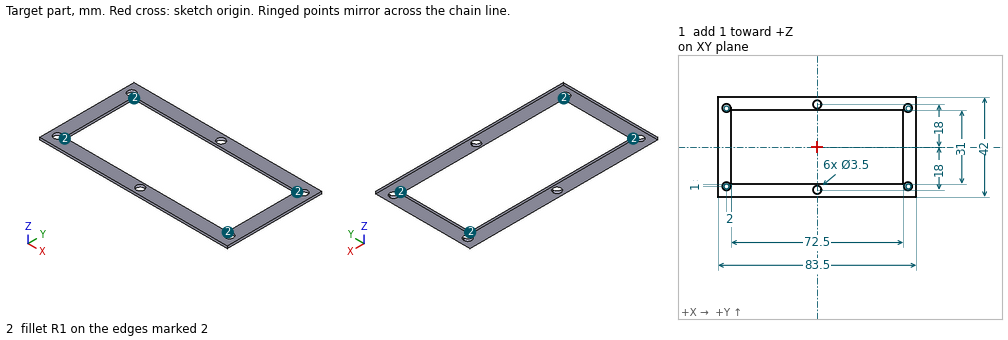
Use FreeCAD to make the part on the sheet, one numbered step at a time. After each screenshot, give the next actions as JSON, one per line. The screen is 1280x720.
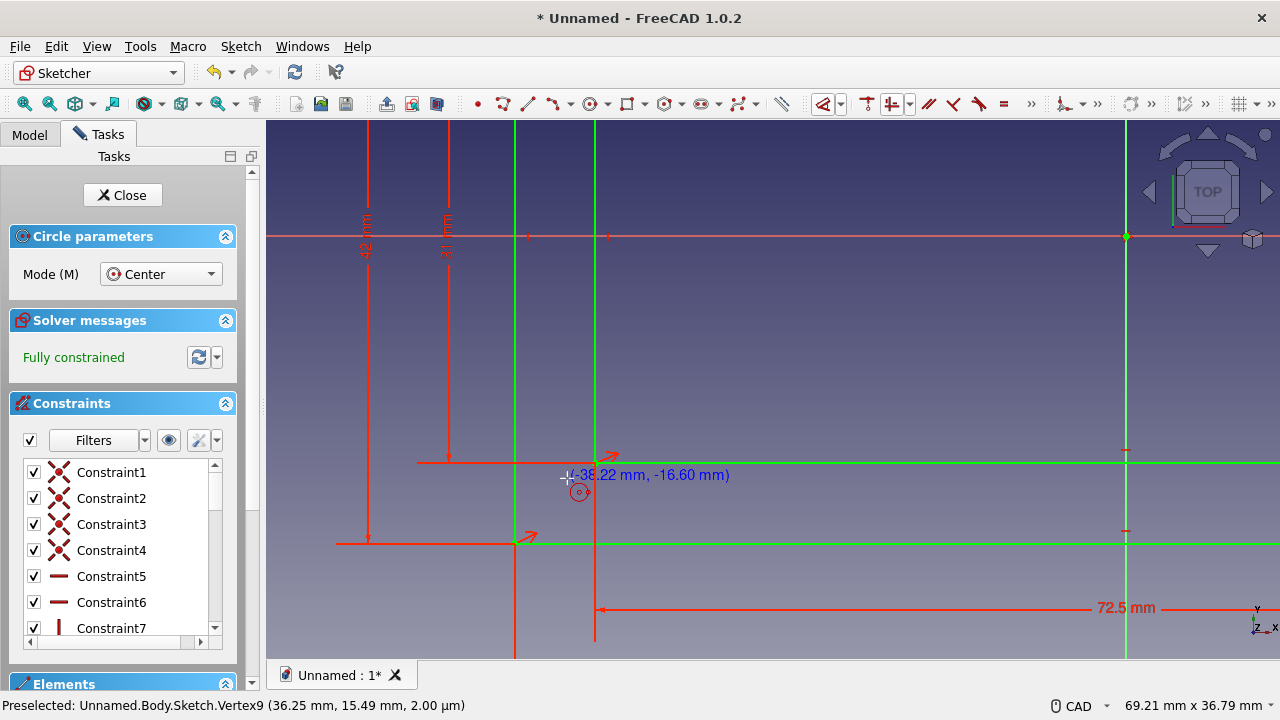
{"action": "left_click", "coordinate": [566, 478]}
{"action": "mouse_move", "coordinate": [548, 460]}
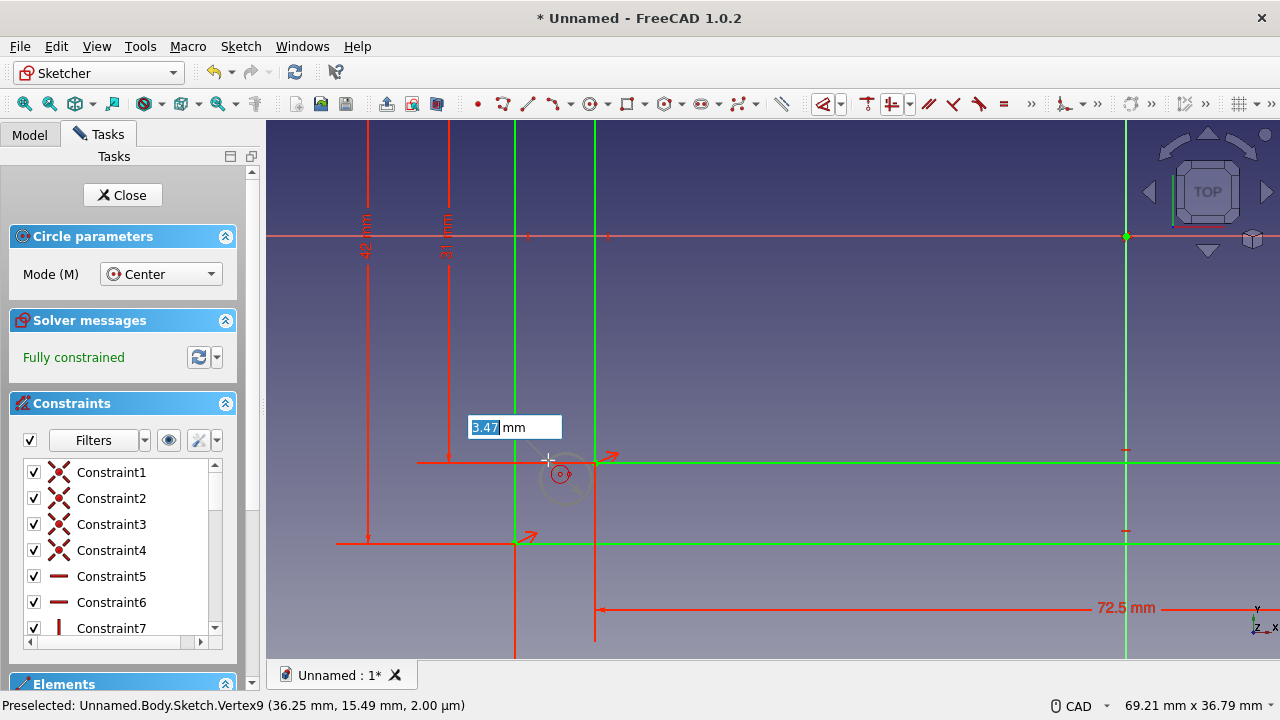
{"action": "type", "text": "3.5"}
{"action": "key", "text": "Return"}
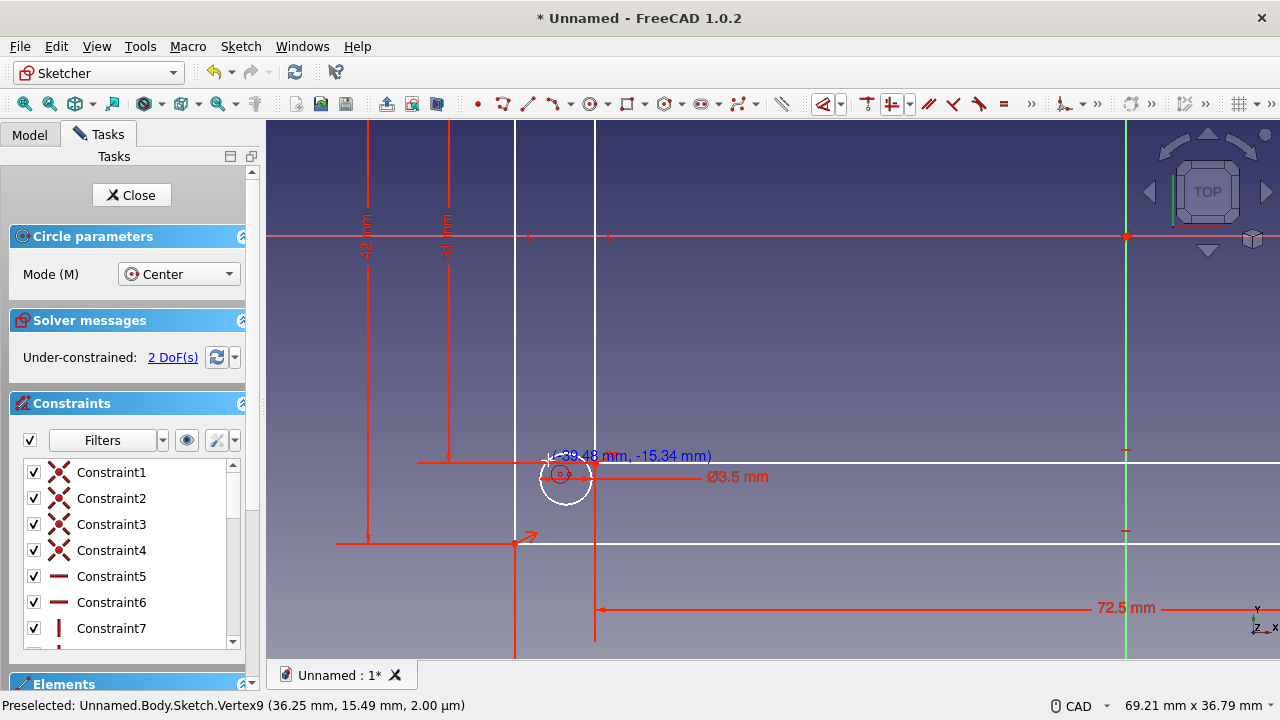
{"action": "scroll", "coordinate": [360, 515], "scroll_direction": "down", "scroll_amount": 4}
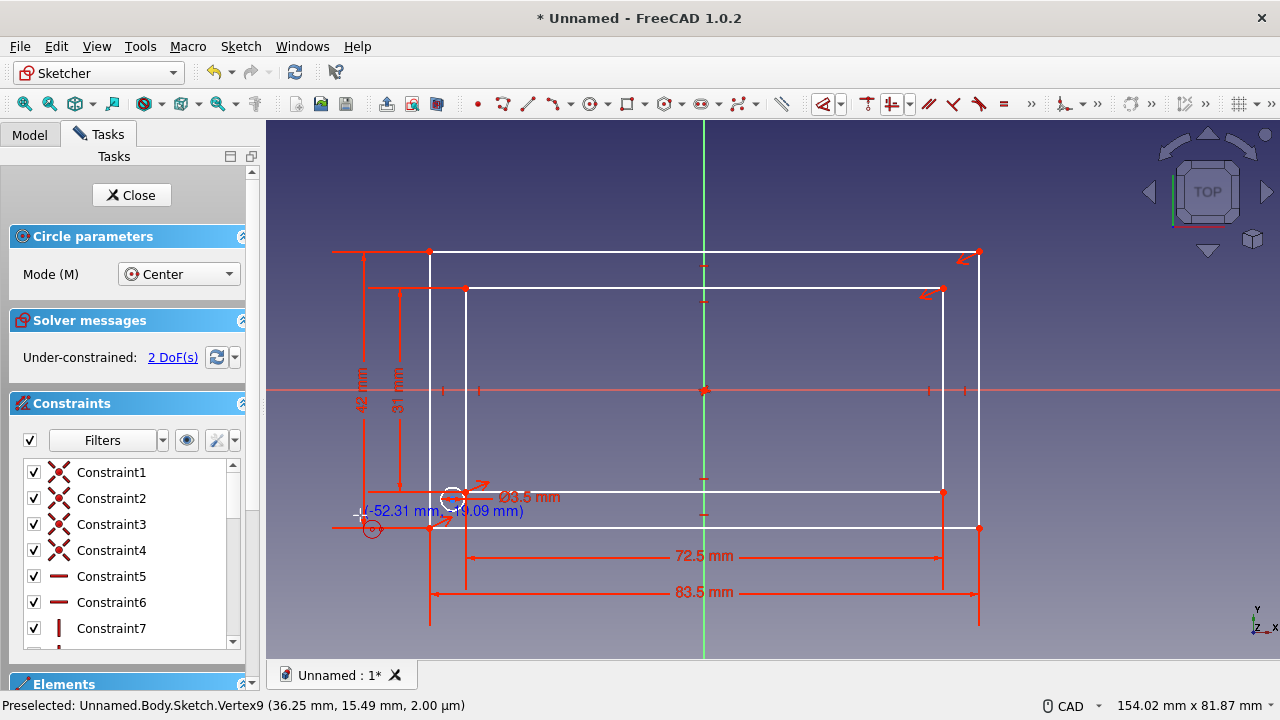
{"action": "scroll", "coordinate": [704, 509], "scroll_direction": "up", "scroll_amount": 4}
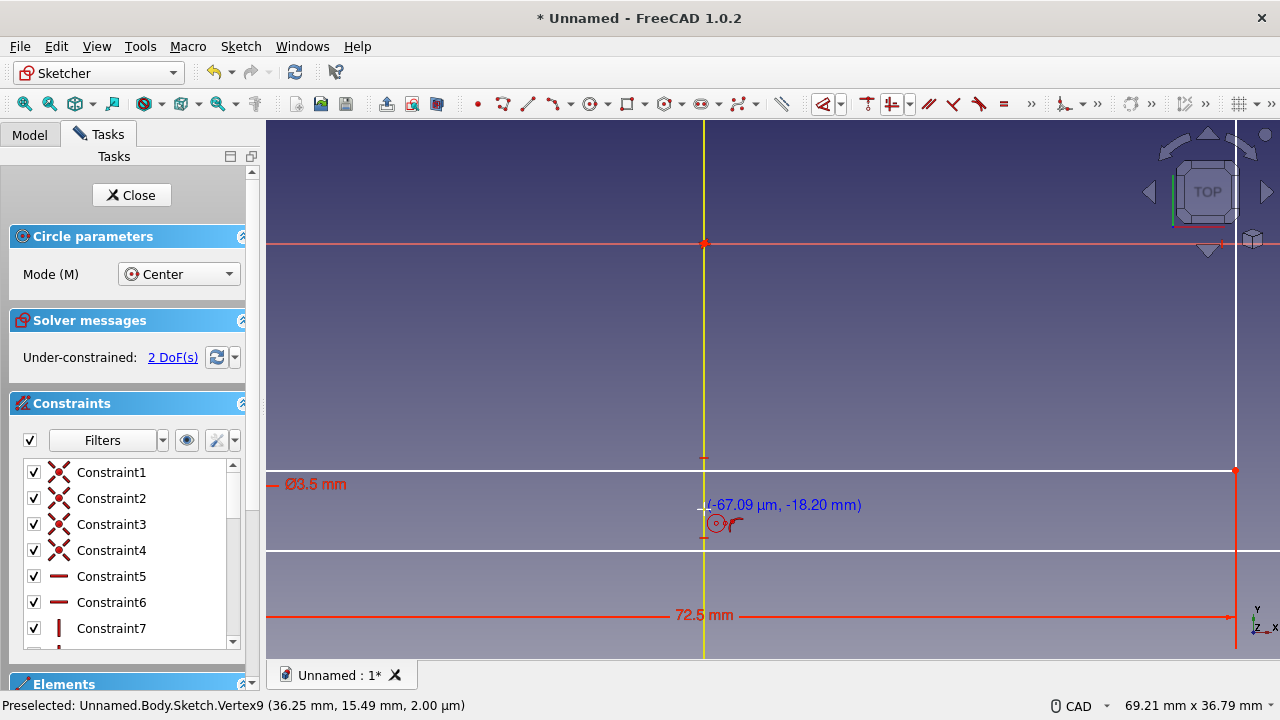
{"action": "left_click", "coordinate": [704, 507]}
{"action": "mouse_move", "coordinate": [723, 489]}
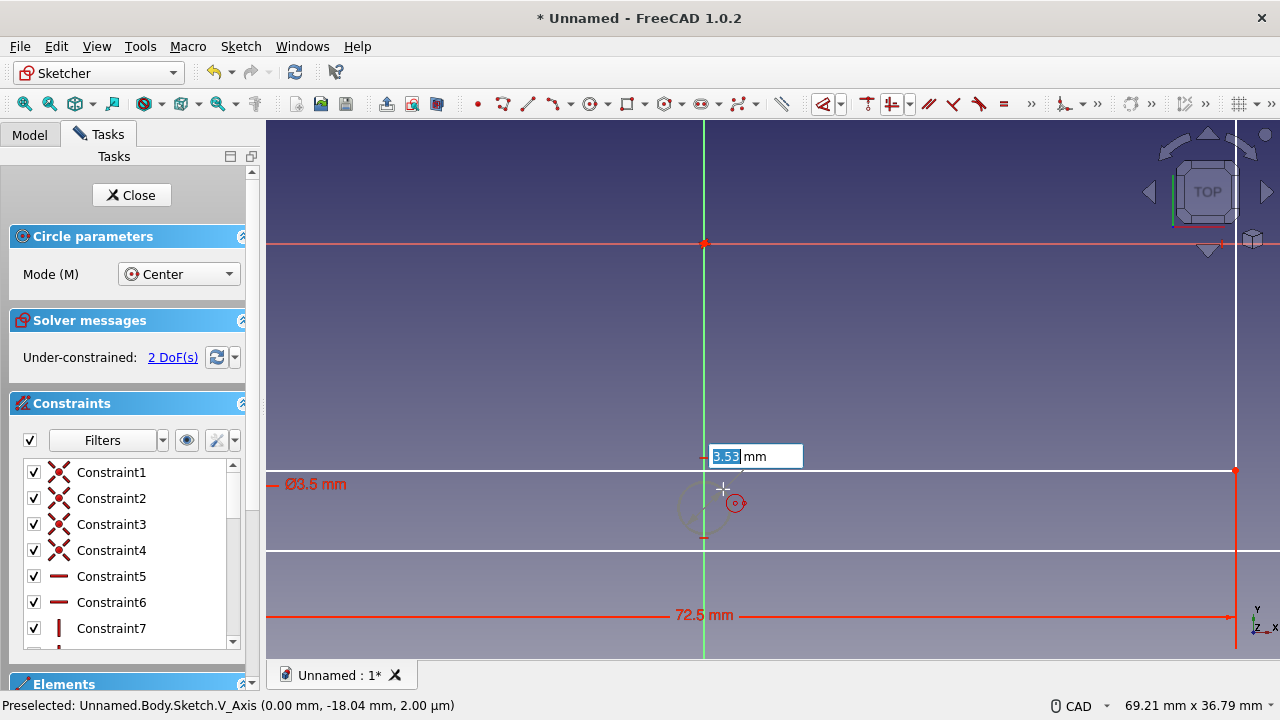
{"action": "type", "text": "3.5"}
{"action": "key", "text": "Return"}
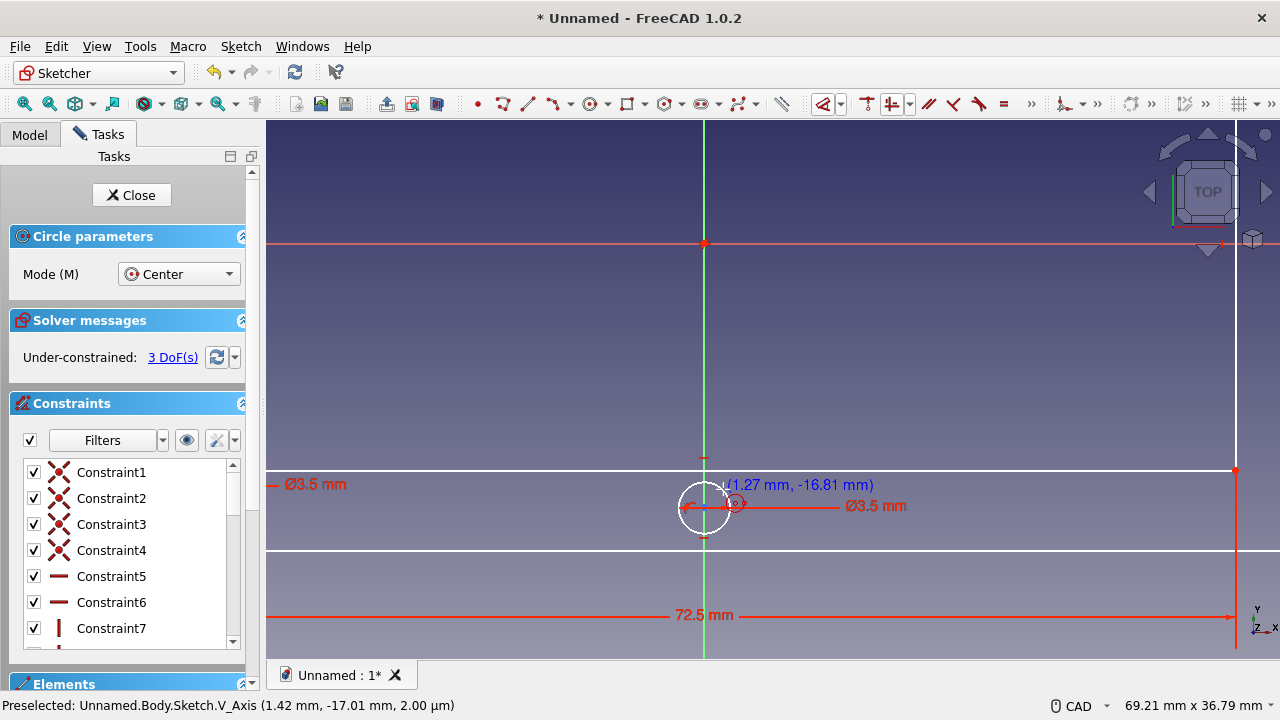
{"action": "scroll", "coordinate": [705, 509], "scroll_direction": "down", "scroll_amount": 4}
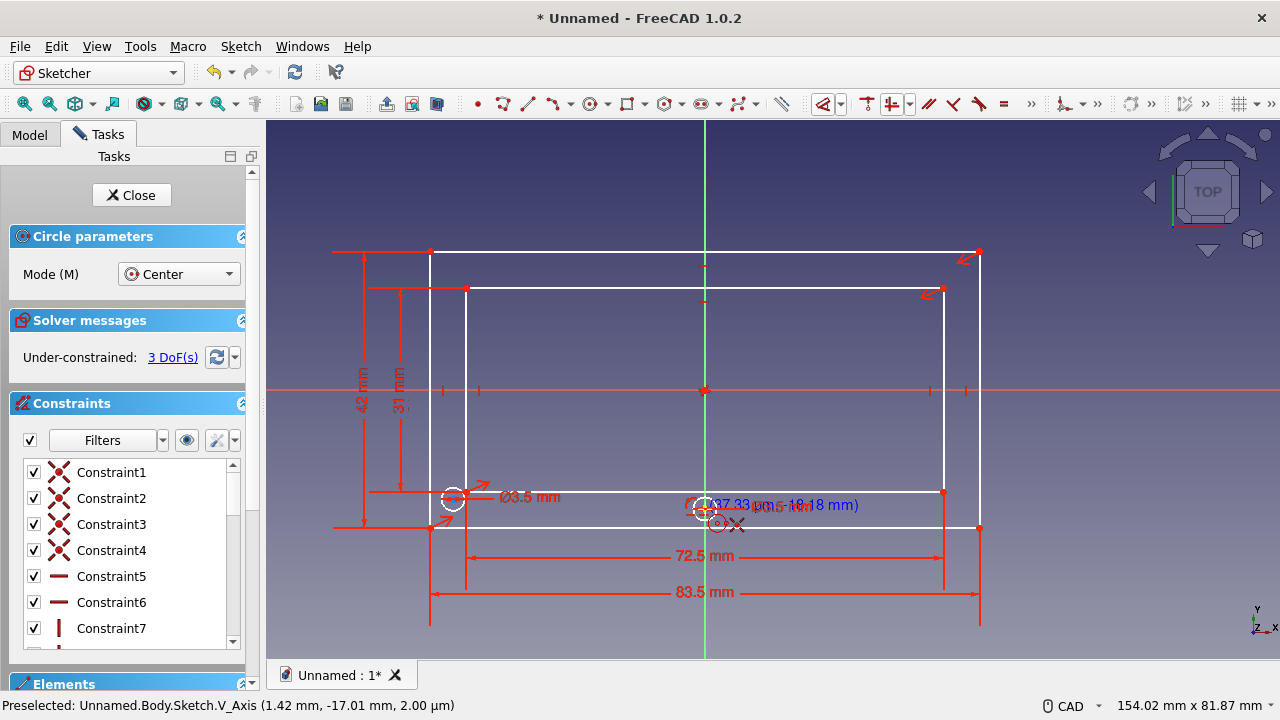
{"action": "scroll", "coordinate": [957, 499], "scroll_direction": "up", "scroll_amount": 4}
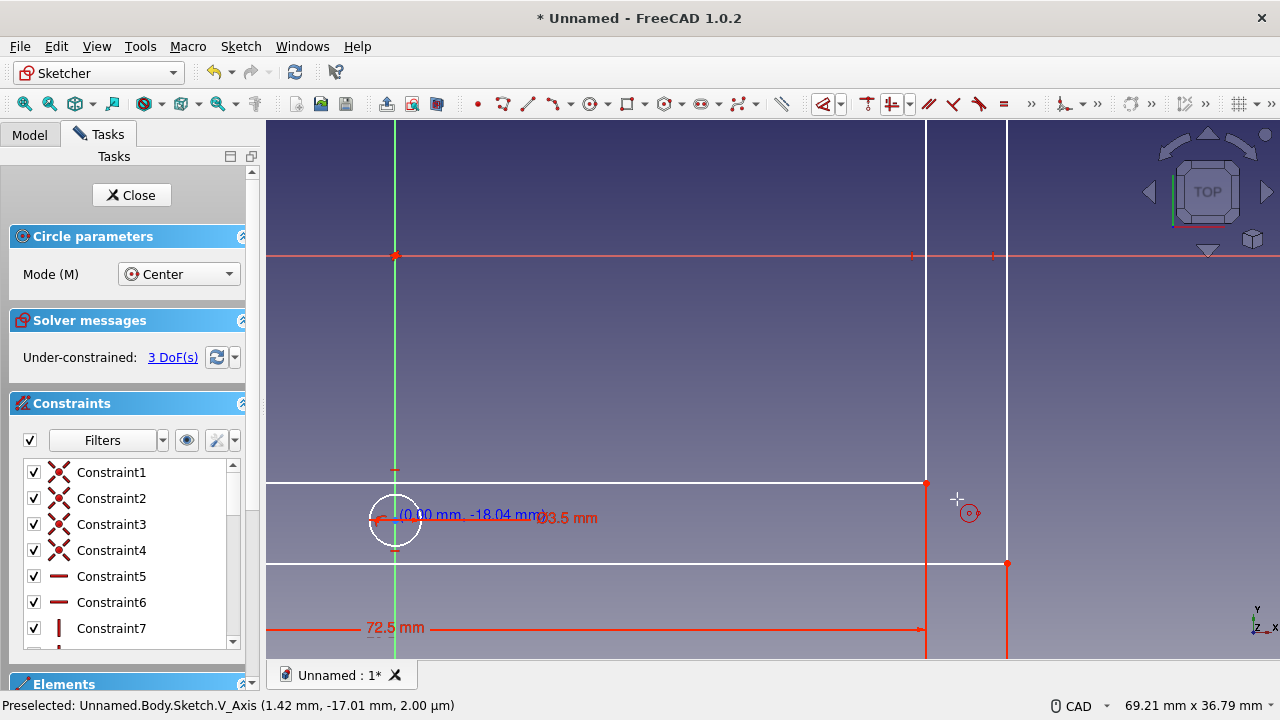
{"action": "left_click", "coordinate": [956, 498]}
{"action": "mouse_move", "coordinate": [974, 480]}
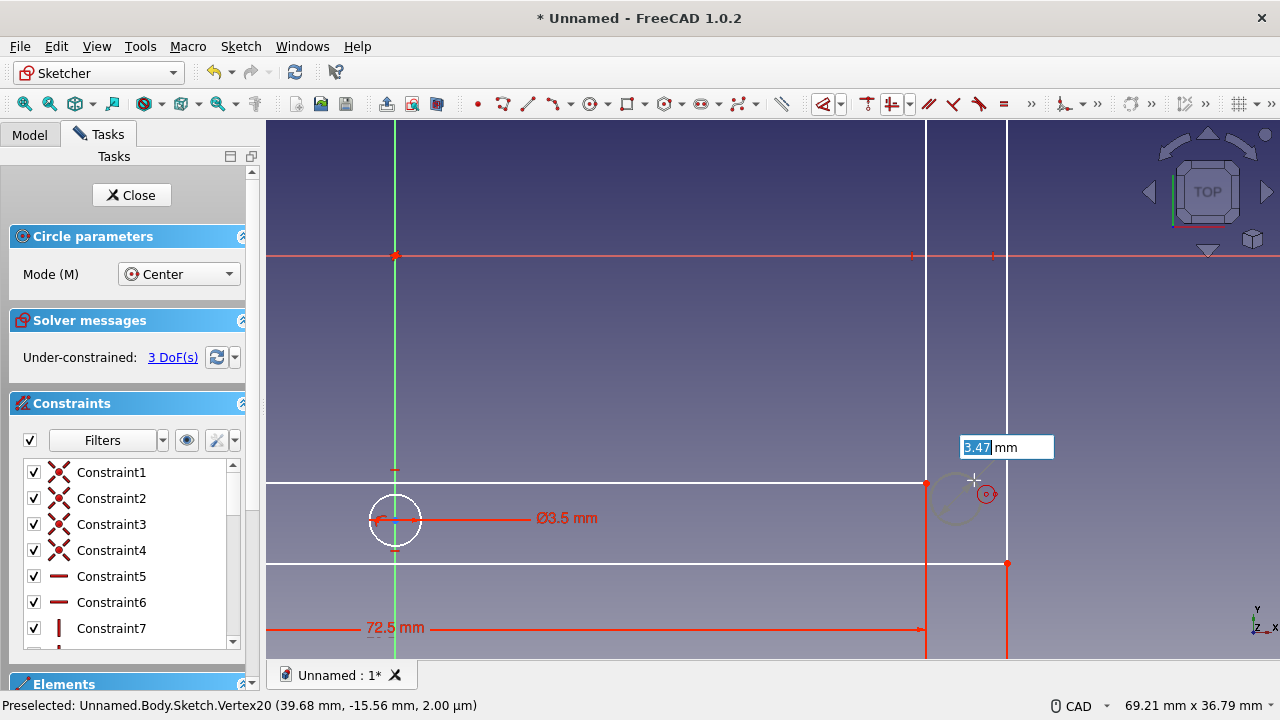
{"action": "type", "text": "3.5"}
{"action": "key", "text": "Return"}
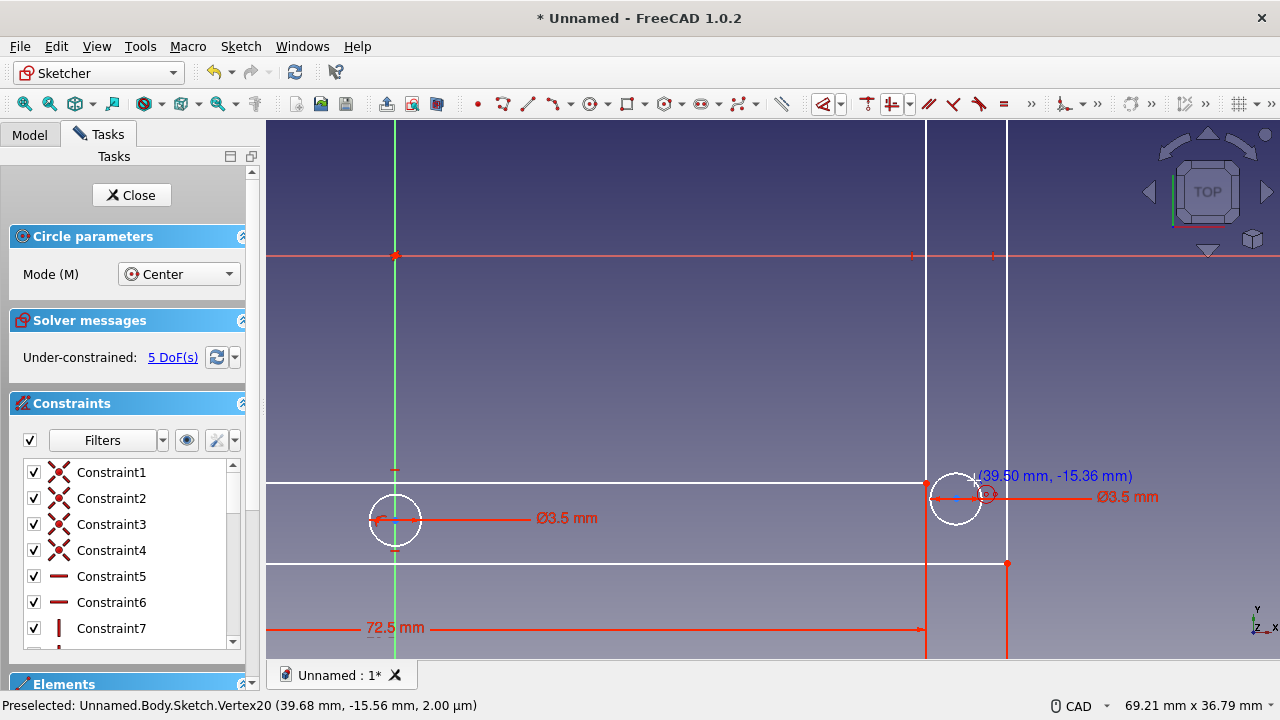
{"action": "scroll", "coordinate": [957, 498], "scroll_direction": "down", "scroll_amount": 4}